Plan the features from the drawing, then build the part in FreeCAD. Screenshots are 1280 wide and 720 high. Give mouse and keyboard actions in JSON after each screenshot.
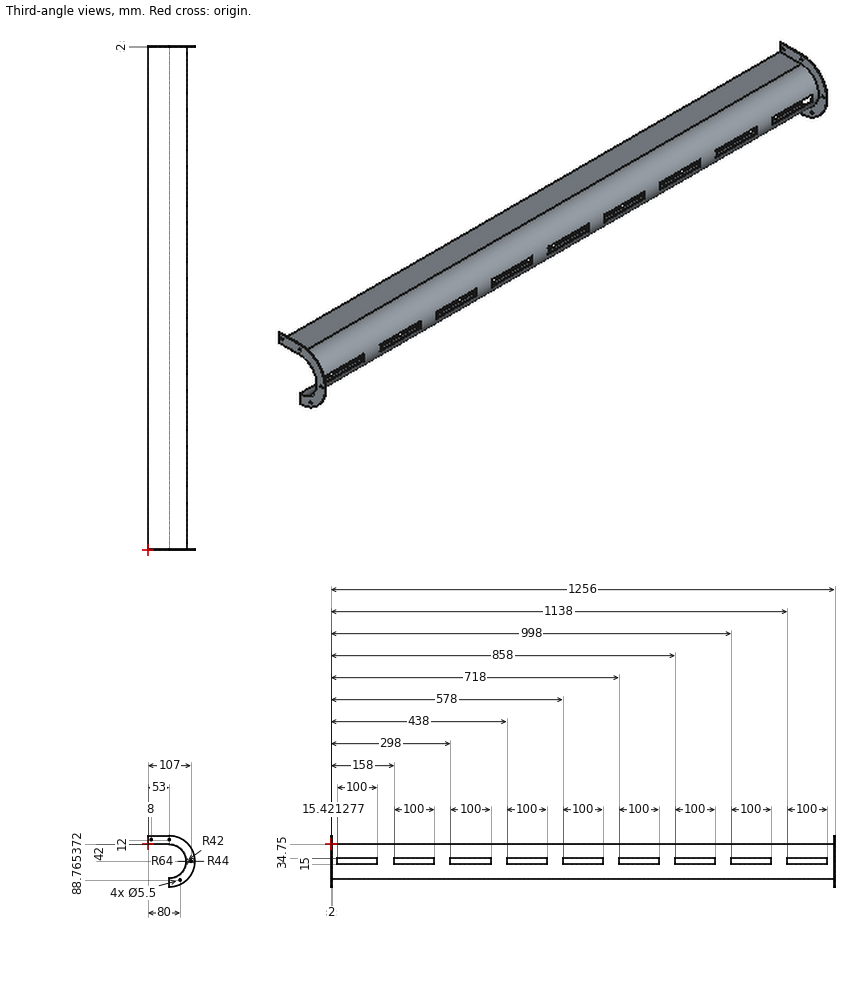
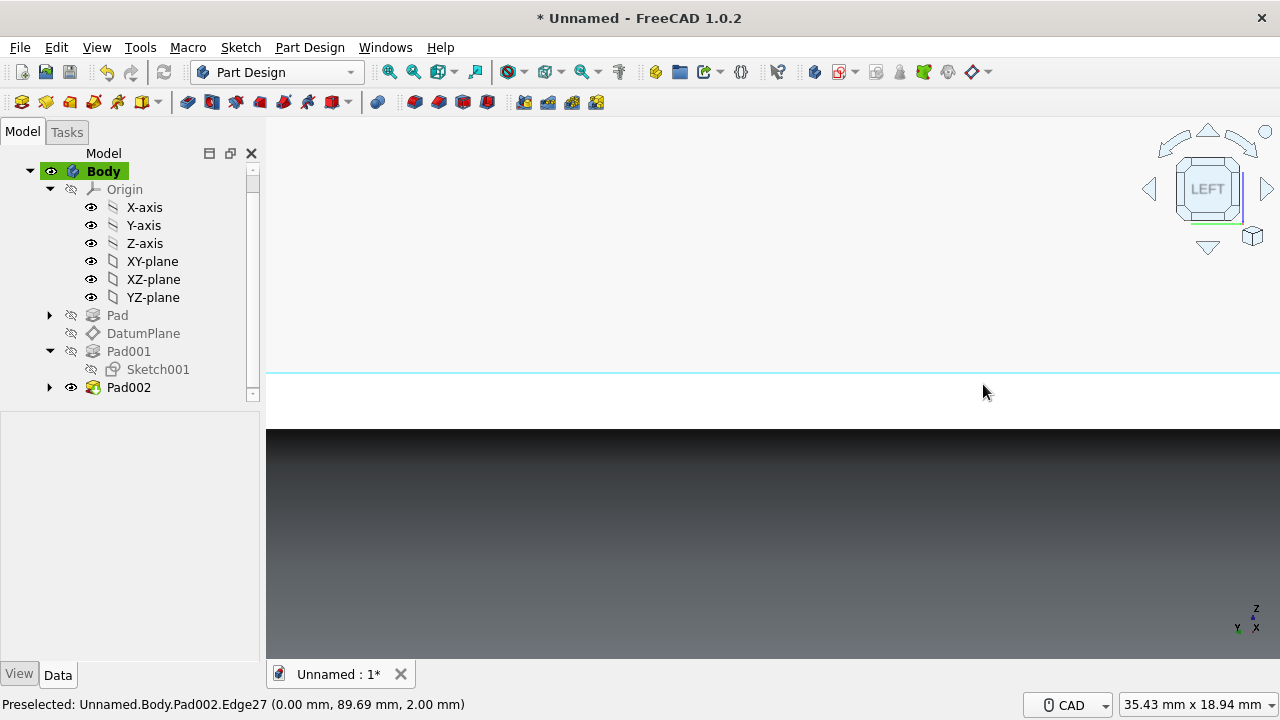
{"action": "left_click", "coordinate": [981, 384]}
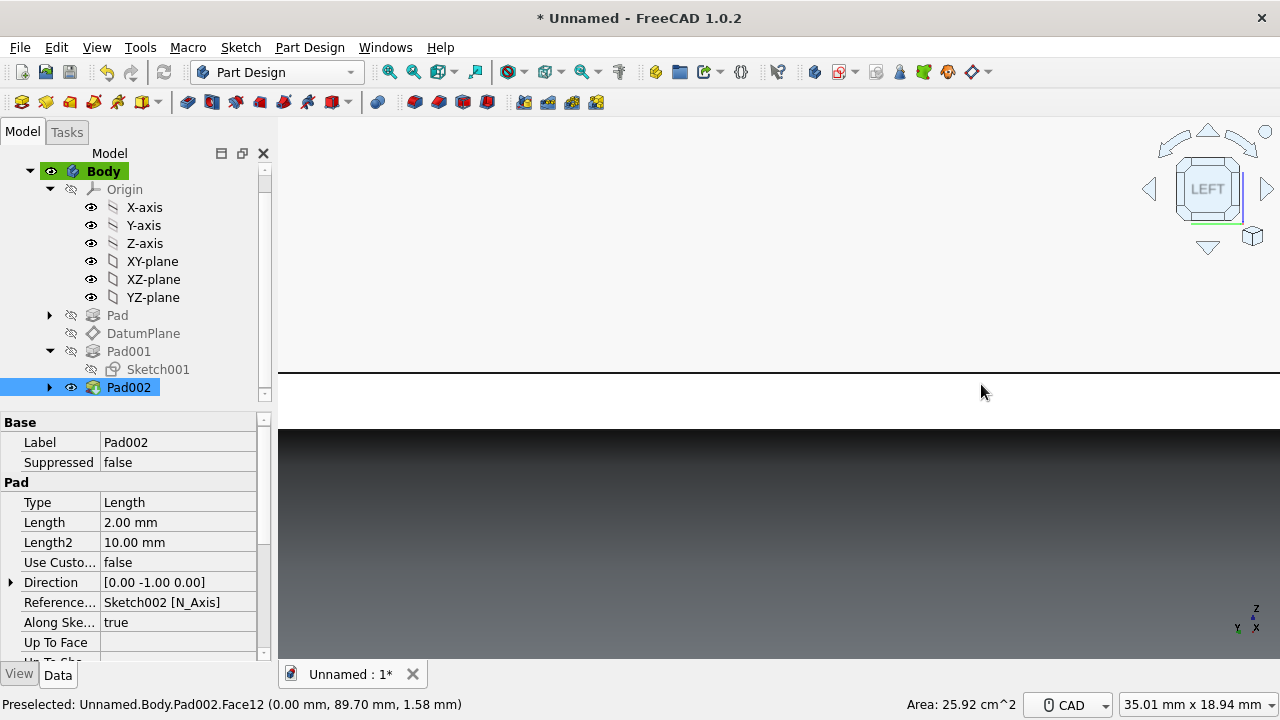
{"action": "left_click", "coordinate": [840, 72]}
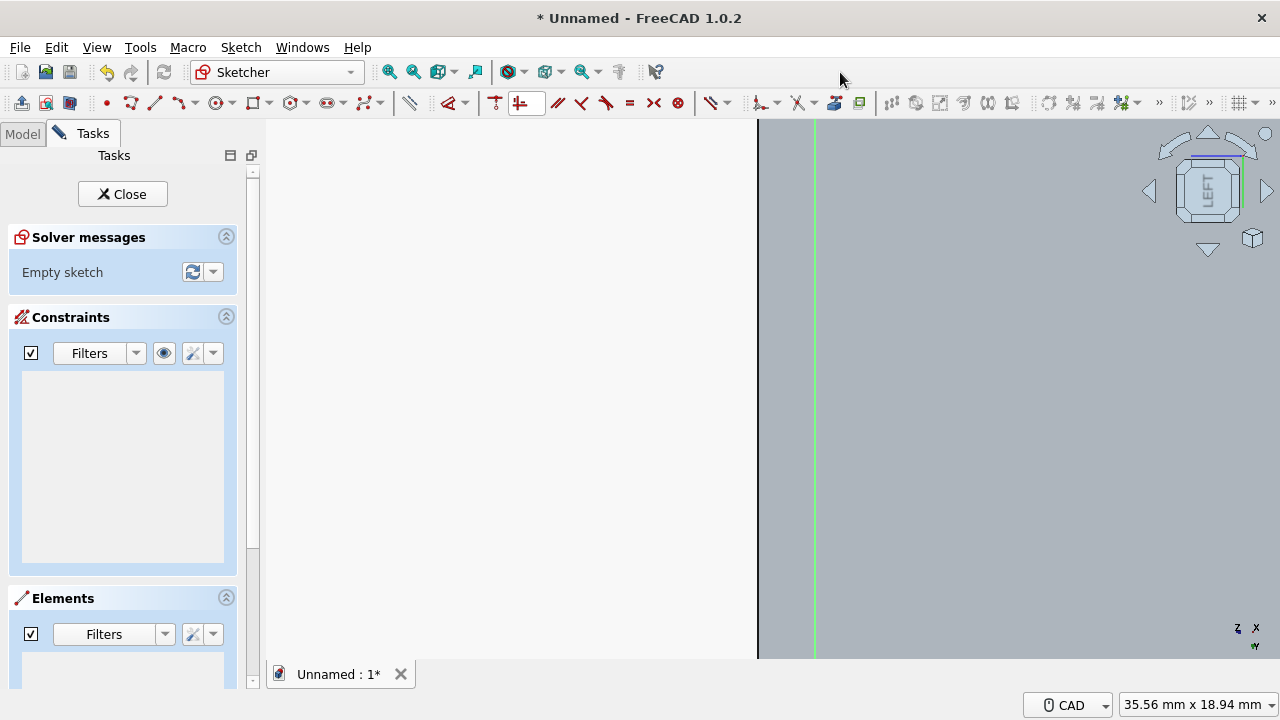
{"action": "scroll", "coordinate": [704, 389], "scroll_direction": "down", "scroll_amount": 15}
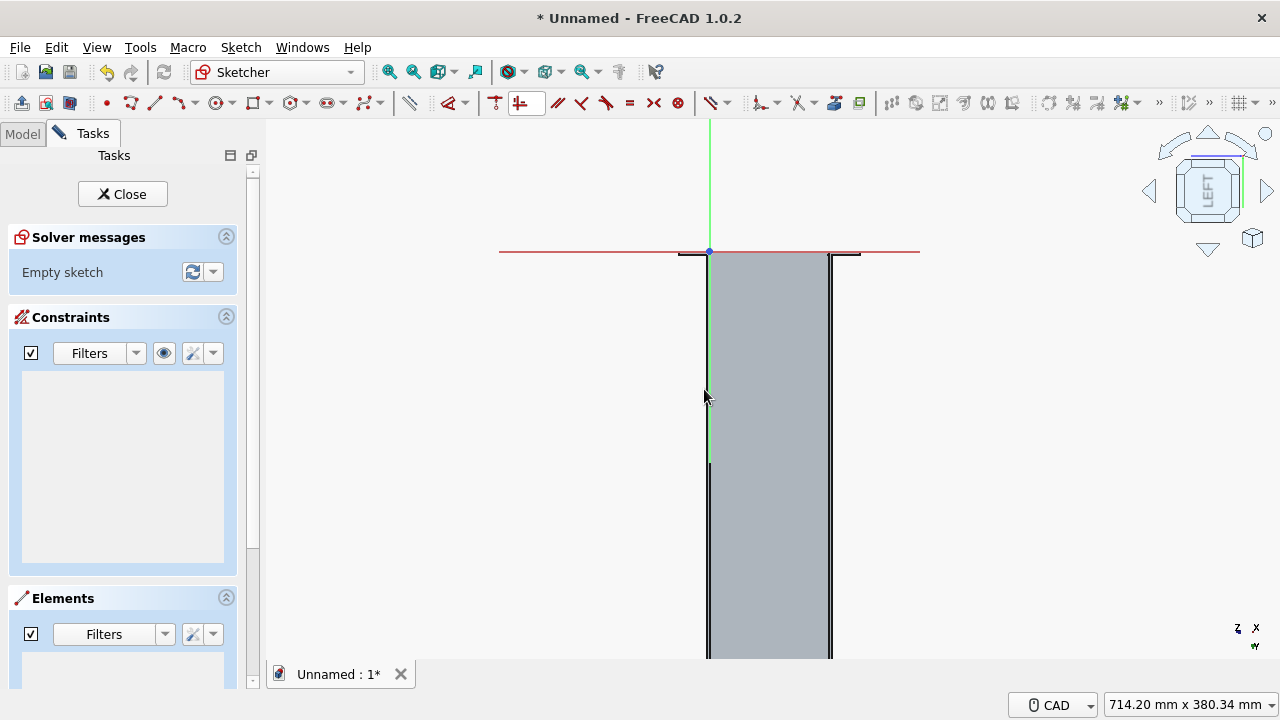
{"action": "scroll", "coordinate": [694, 201], "scroll_direction": "down", "scroll_amount": 8}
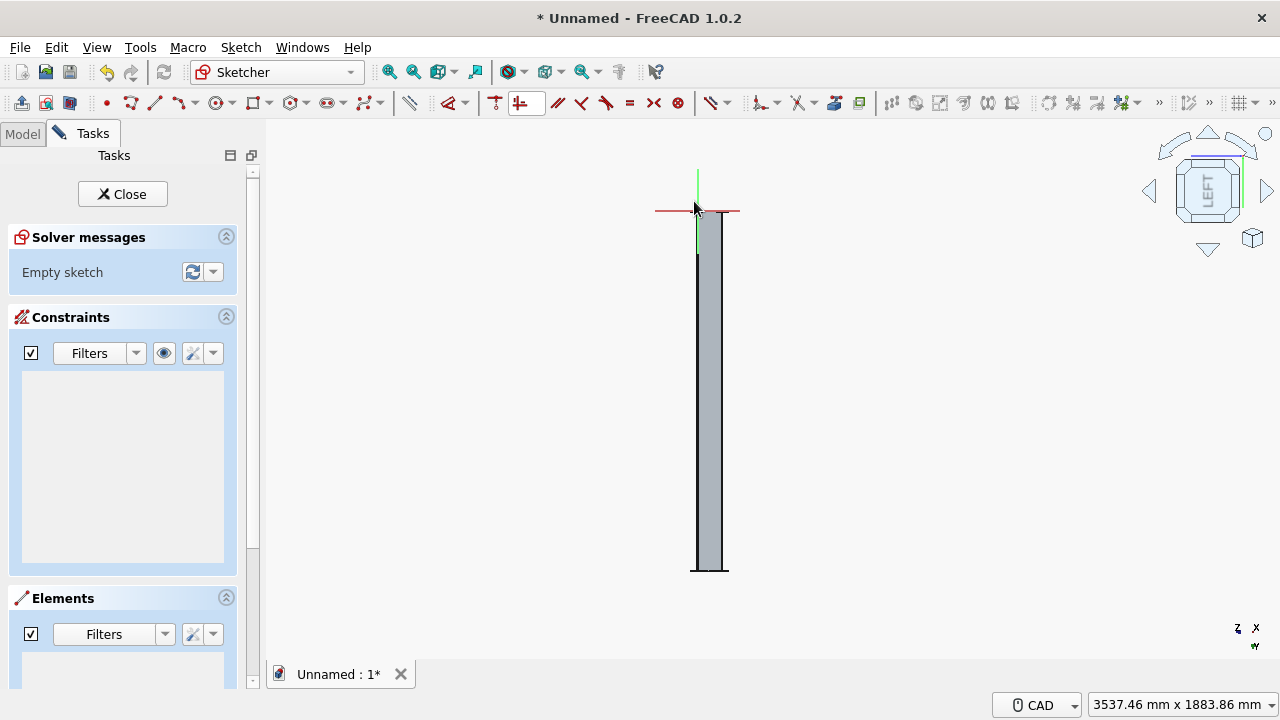
{"action": "left_click", "coordinate": [254, 104]}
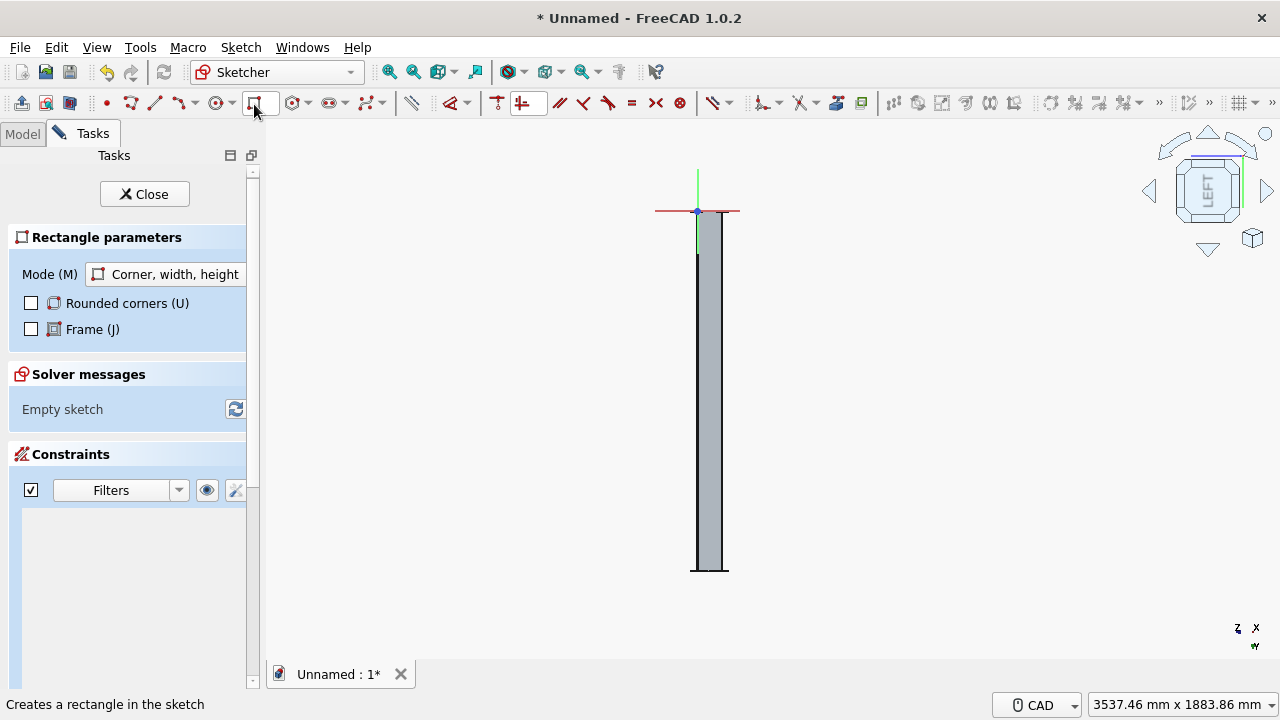
{"action": "scroll", "coordinate": [708, 216], "scroll_direction": "up", "scroll_amount": 7}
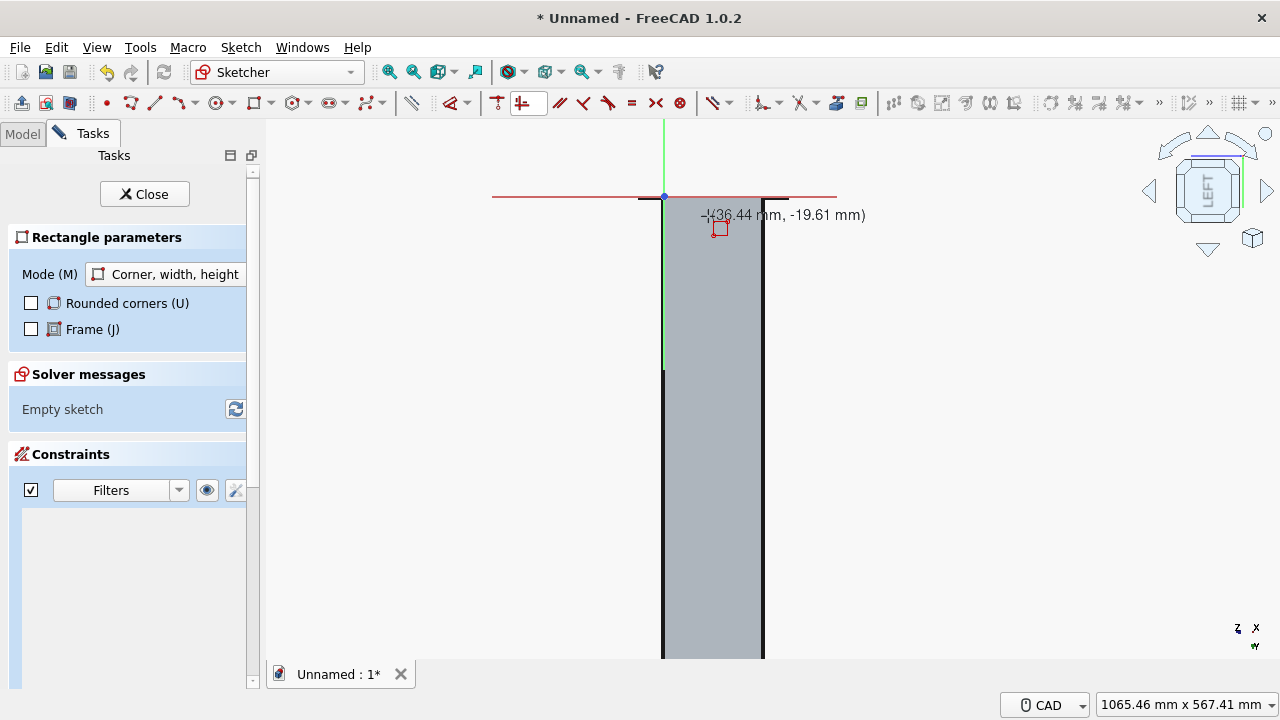
{"action": "left_click", "coordinate": [705, 215]}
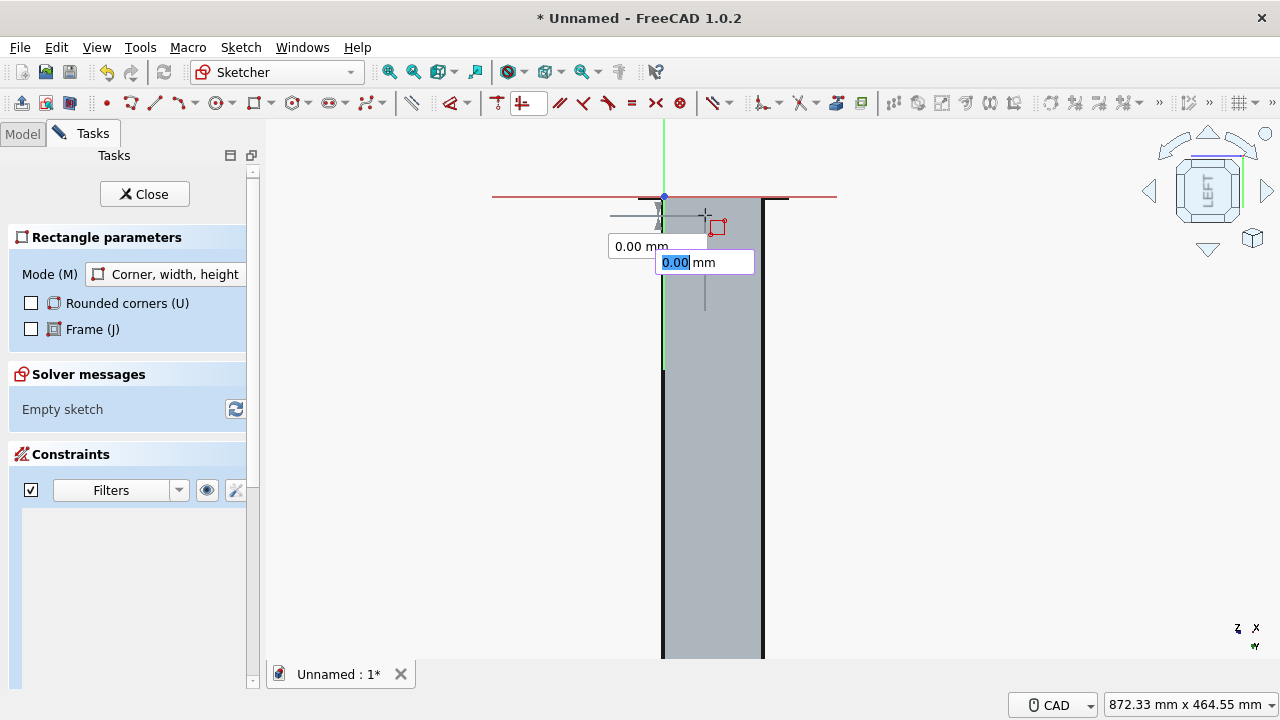
{"action": "scroll", "coordinate": [708, 216], "scroll_direction": "down", "scroll_amount": 7}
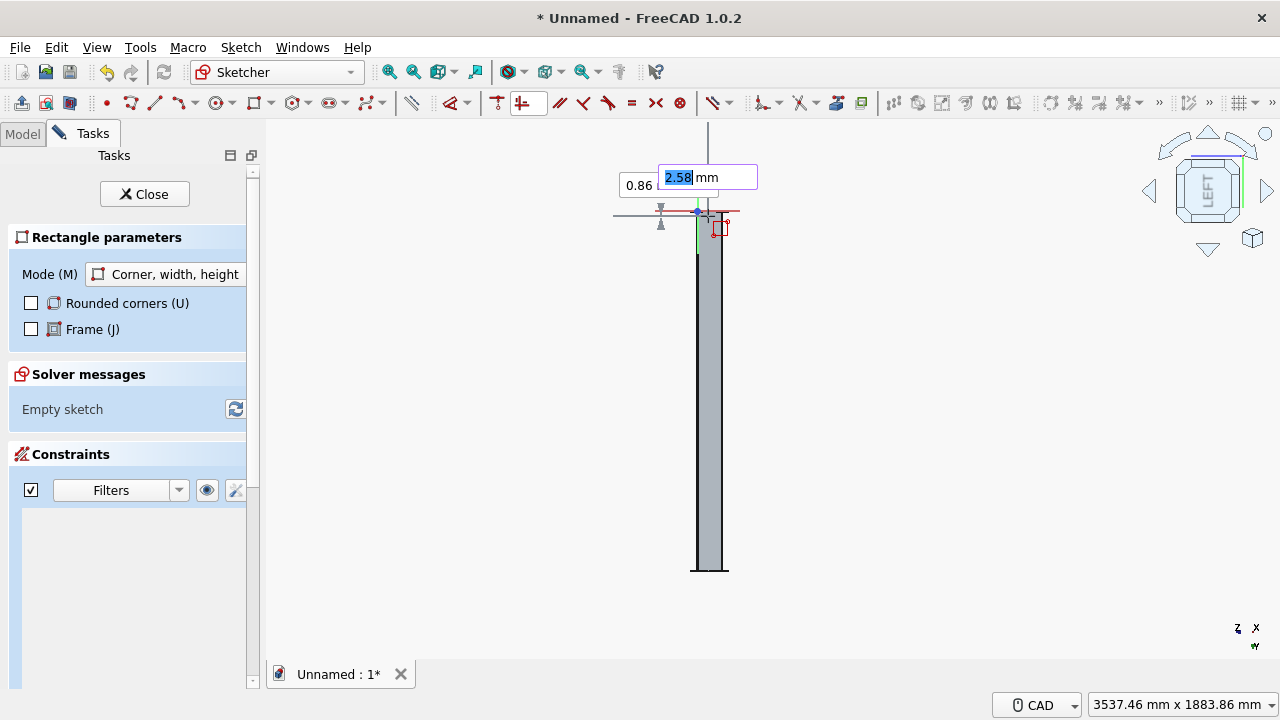
{"action": "left_click", "coordinate": [712, 244]}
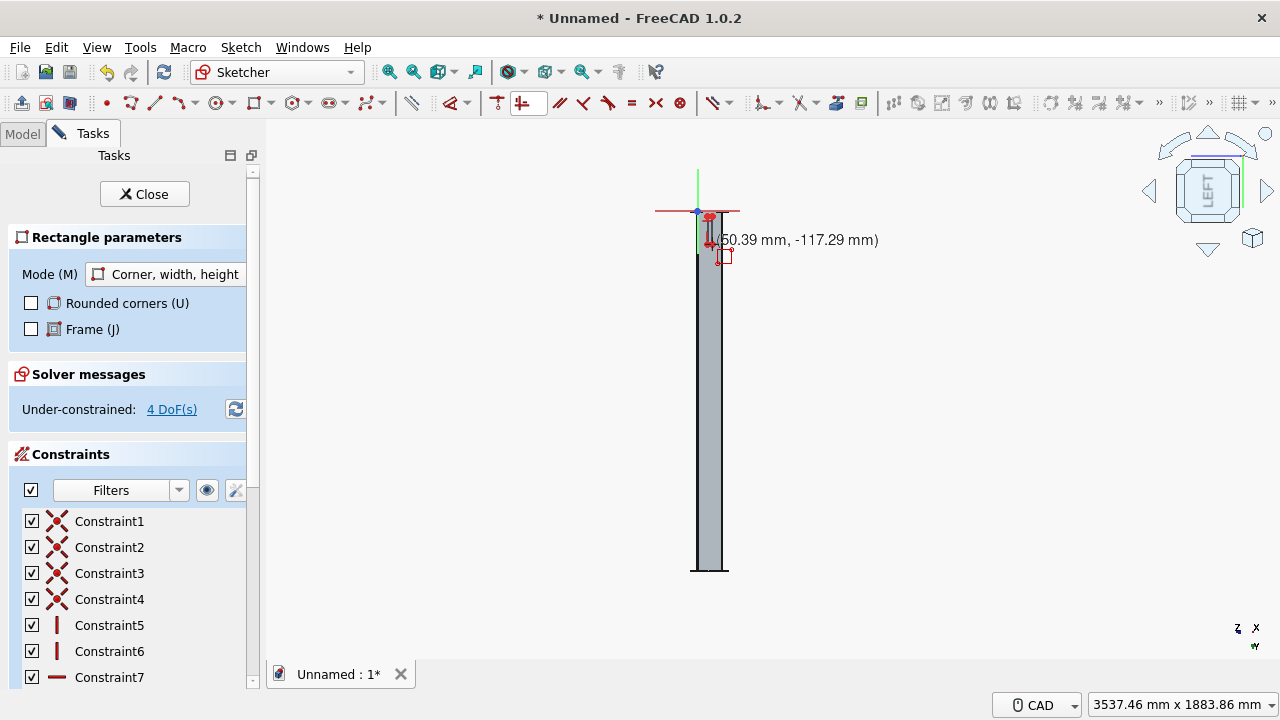
{"action": "scroll", "coordinate": [708, 257], "scroll_direction": "up", "scroll_amount": 7}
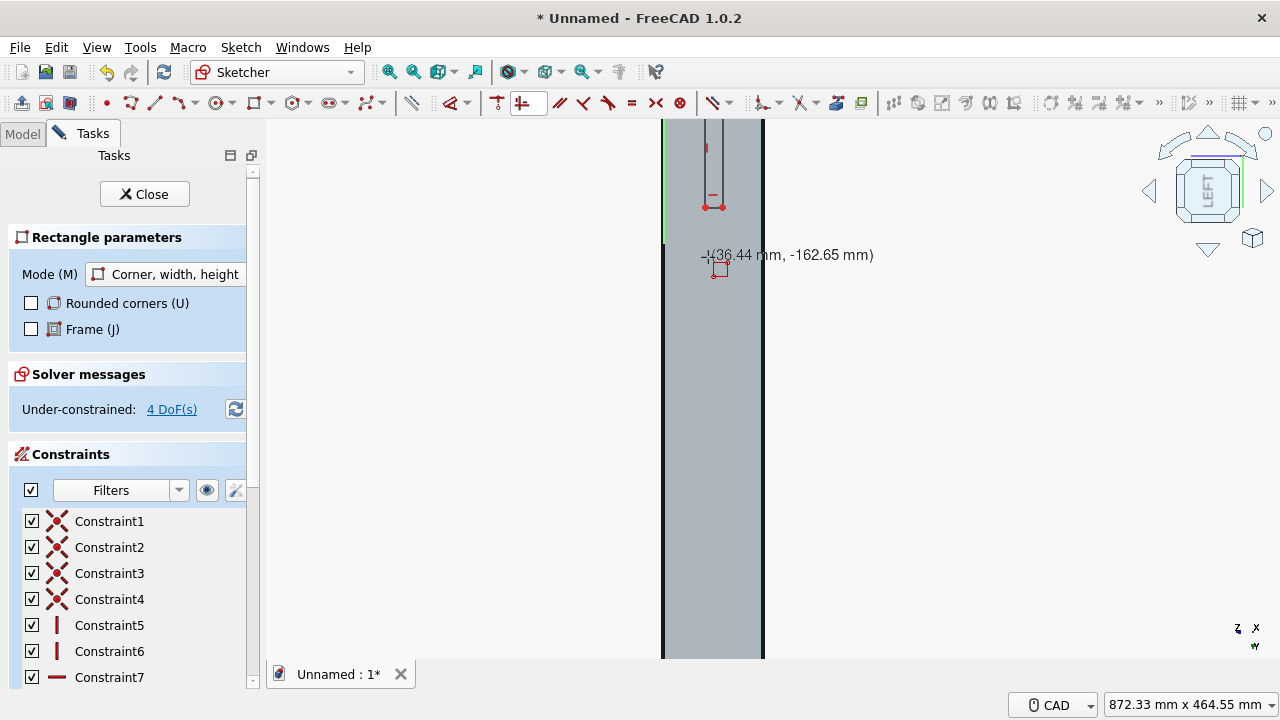
{"action": "left_click", "coordinate": [705, 255]}